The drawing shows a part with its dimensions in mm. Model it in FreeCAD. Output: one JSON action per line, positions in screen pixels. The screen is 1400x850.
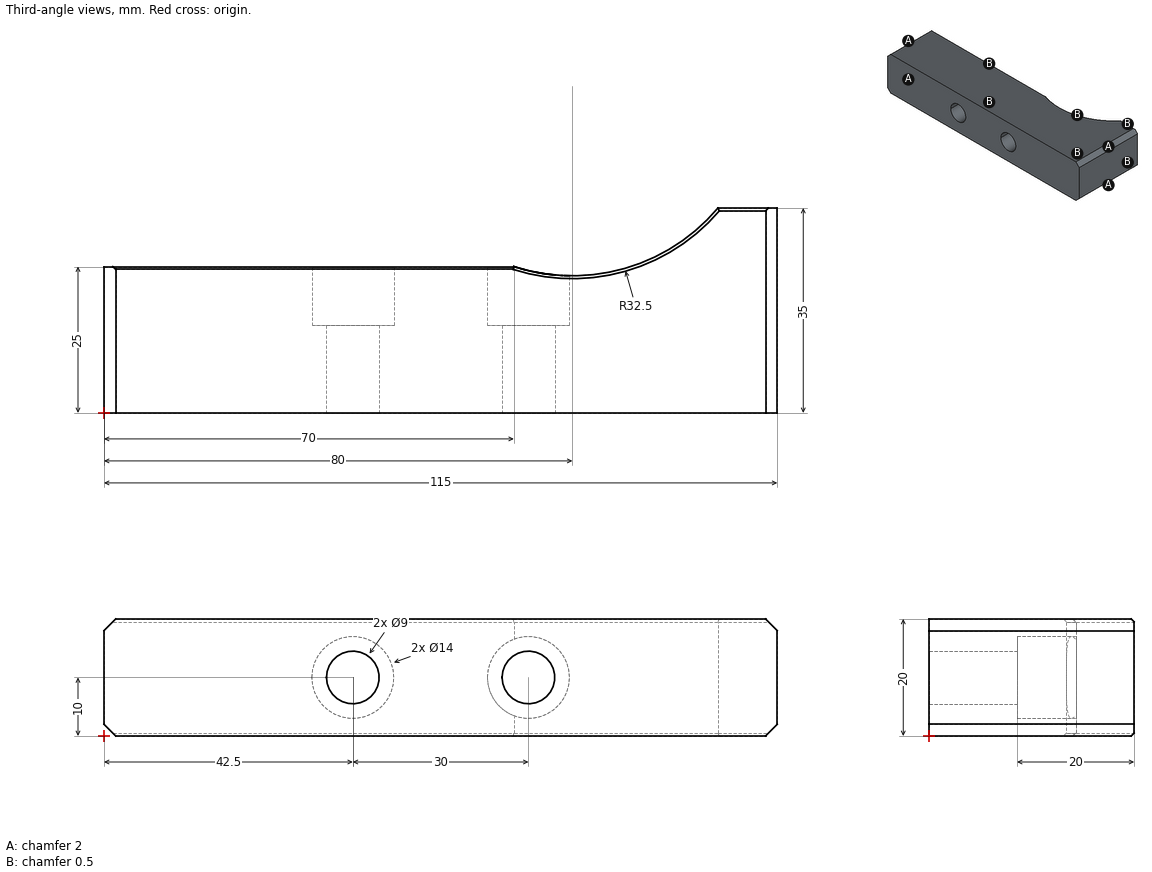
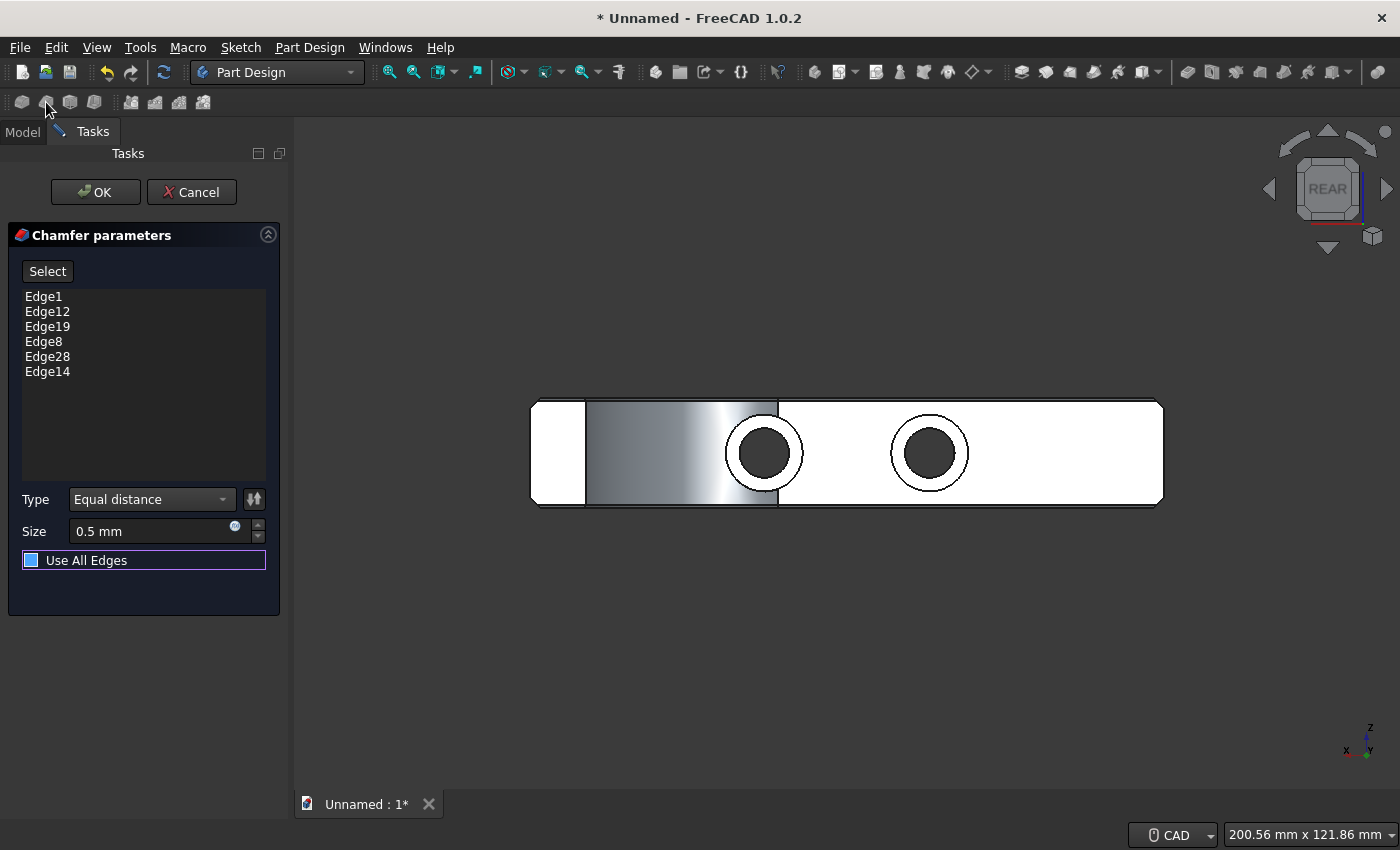
{"action": "left_click", "coordinate": [96, 192]}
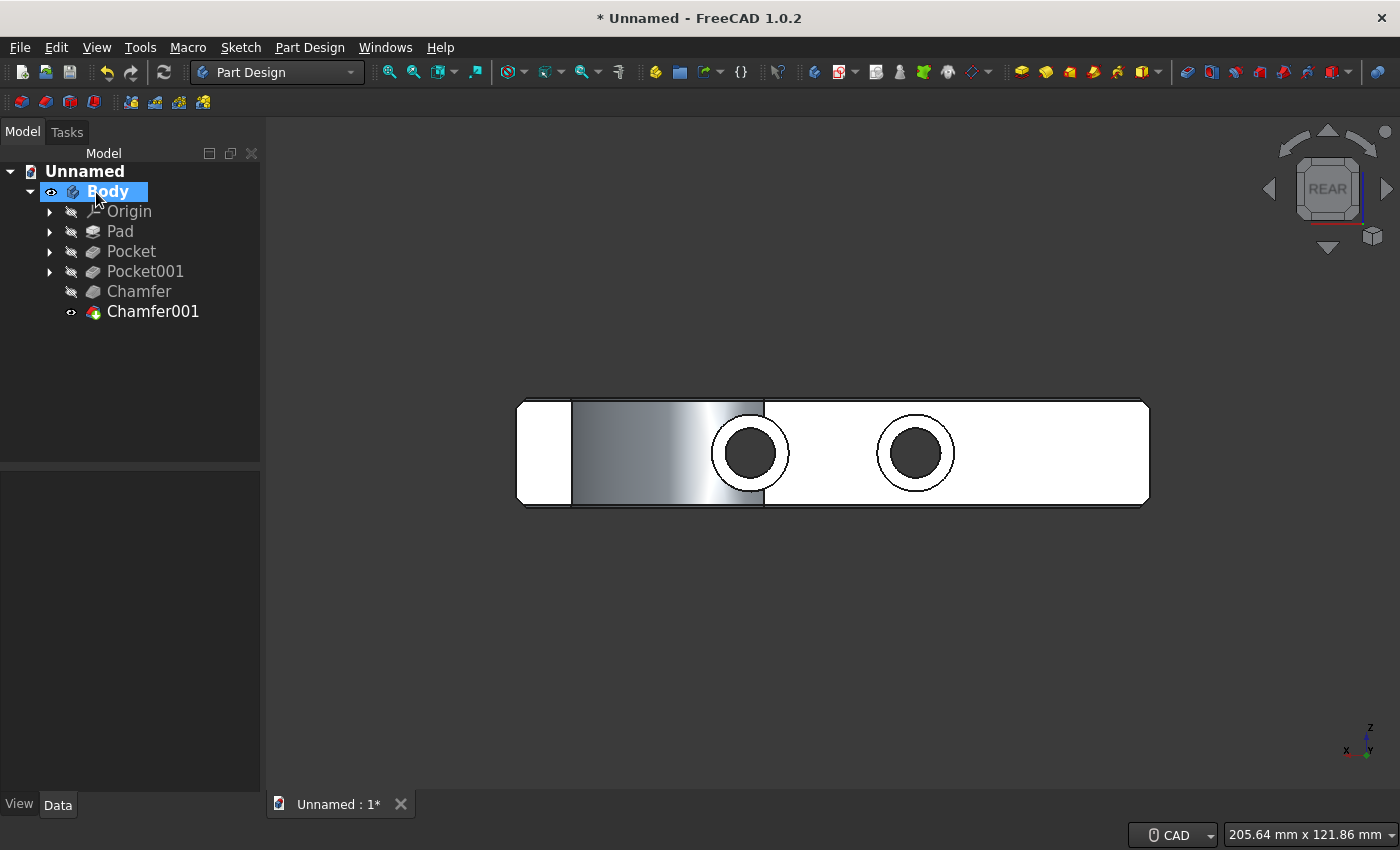
{"action": "key", "text": "0"}